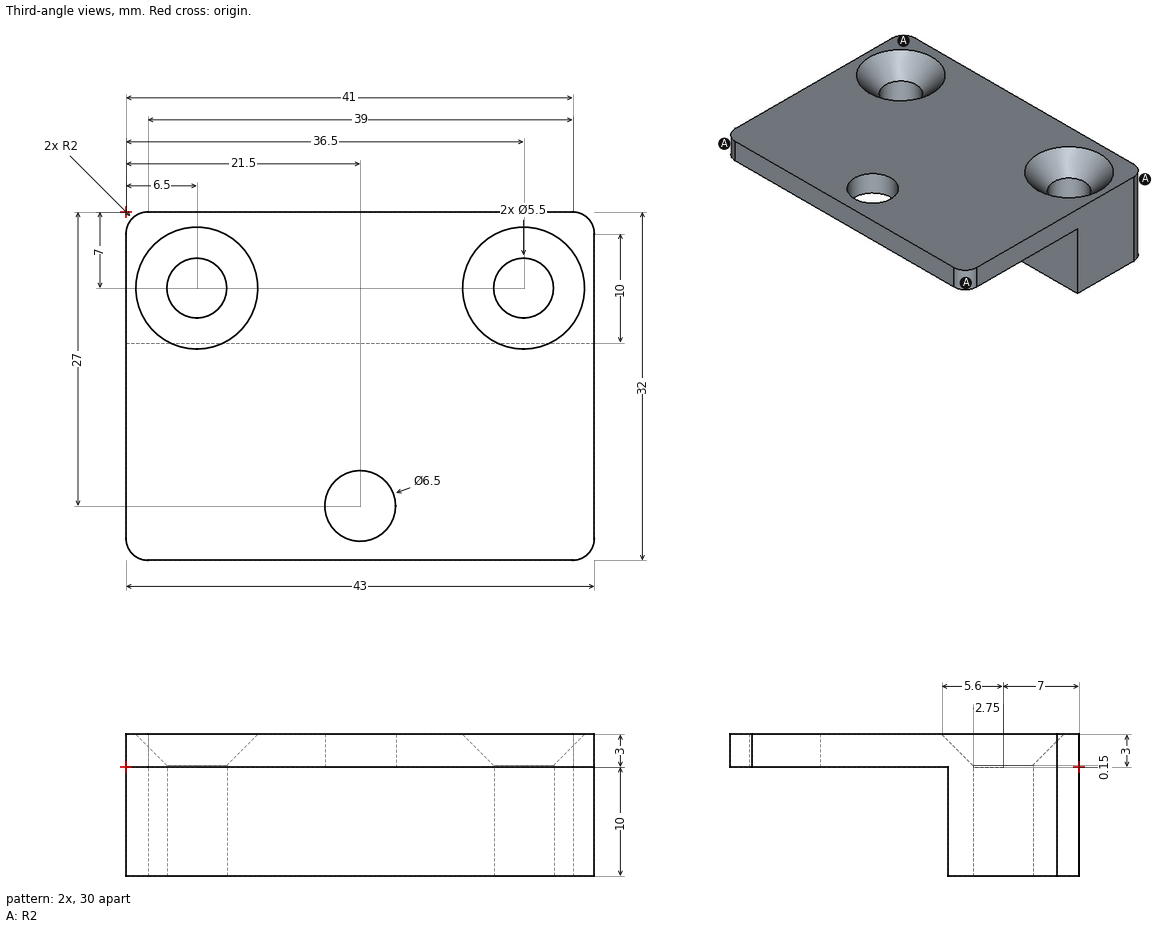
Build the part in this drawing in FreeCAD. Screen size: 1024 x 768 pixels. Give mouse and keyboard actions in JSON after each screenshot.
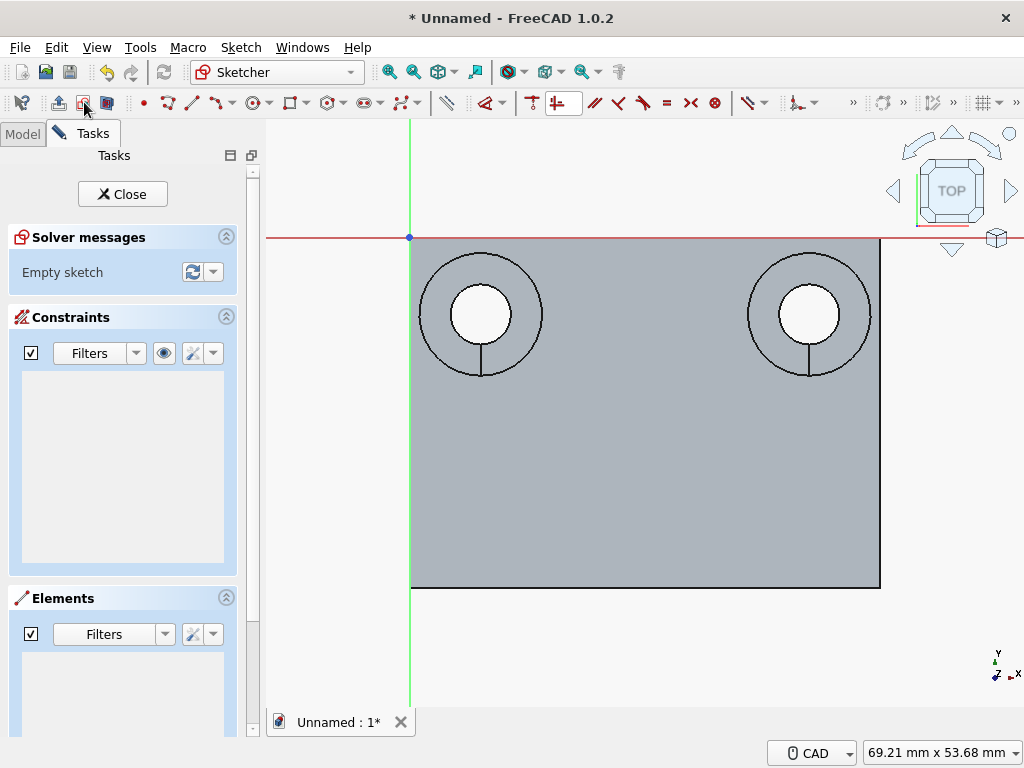
{"action": "scroll", "coordinate": [662, 564], "scroll_direction": "up", "scroll_amount": 8}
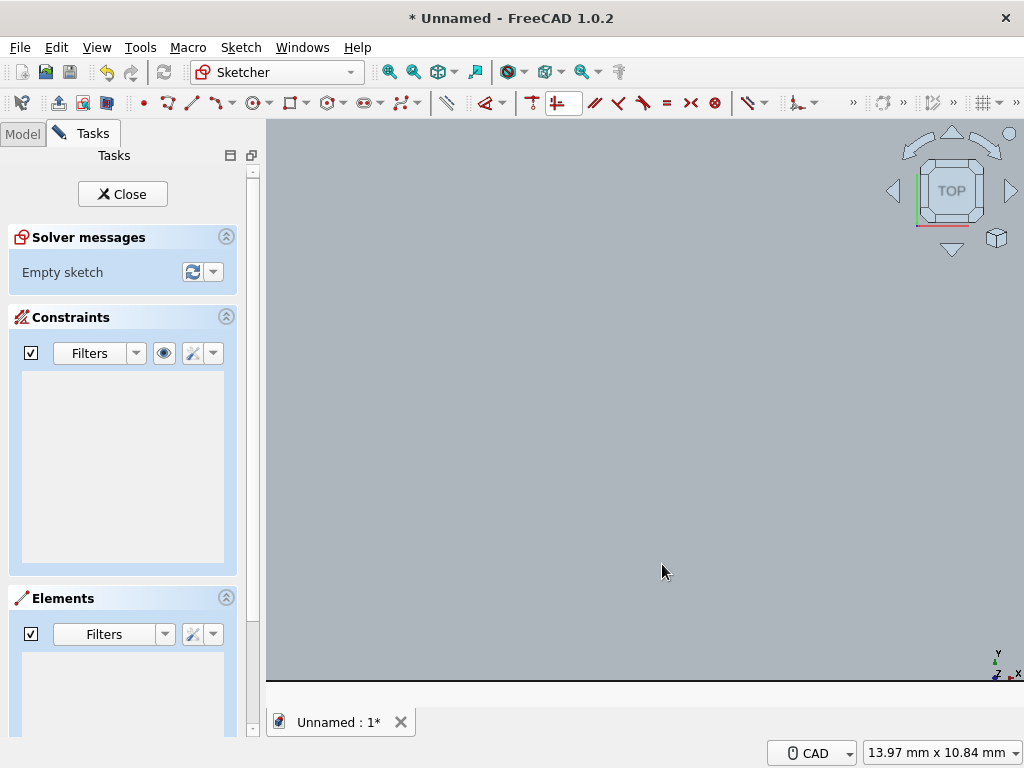
{"action": "key", "text": "g c"}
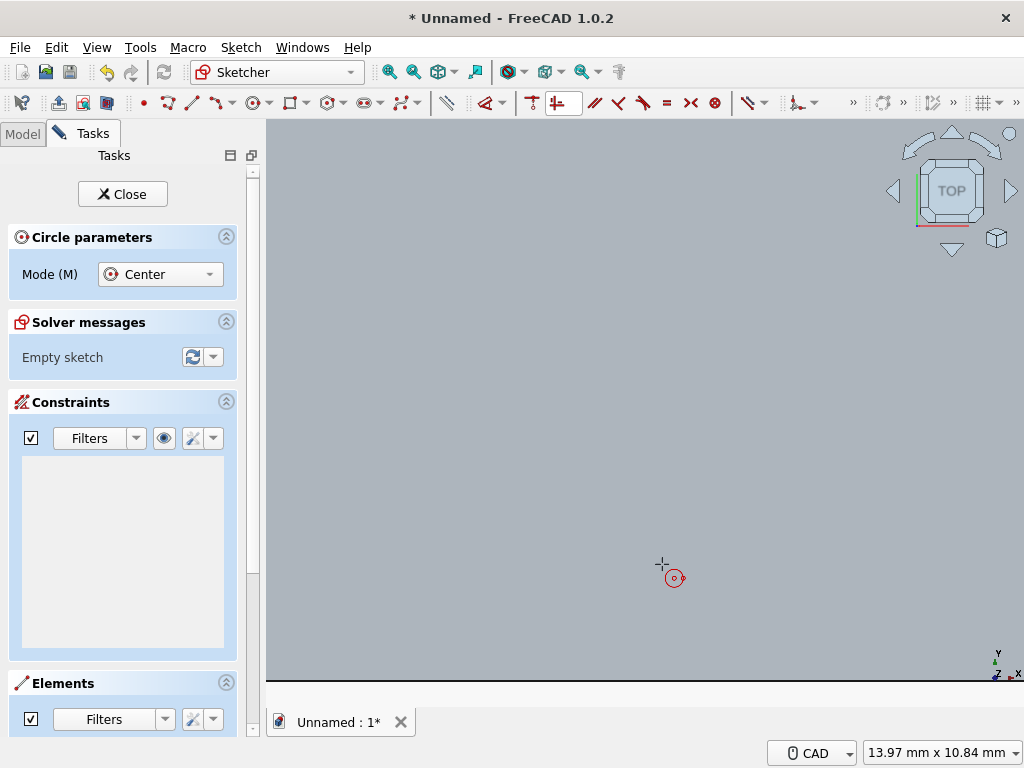
{"action": "left_click", "coordinate": [576, 410]}
{"action": "mouse_move", "coordinate": [700, 285]}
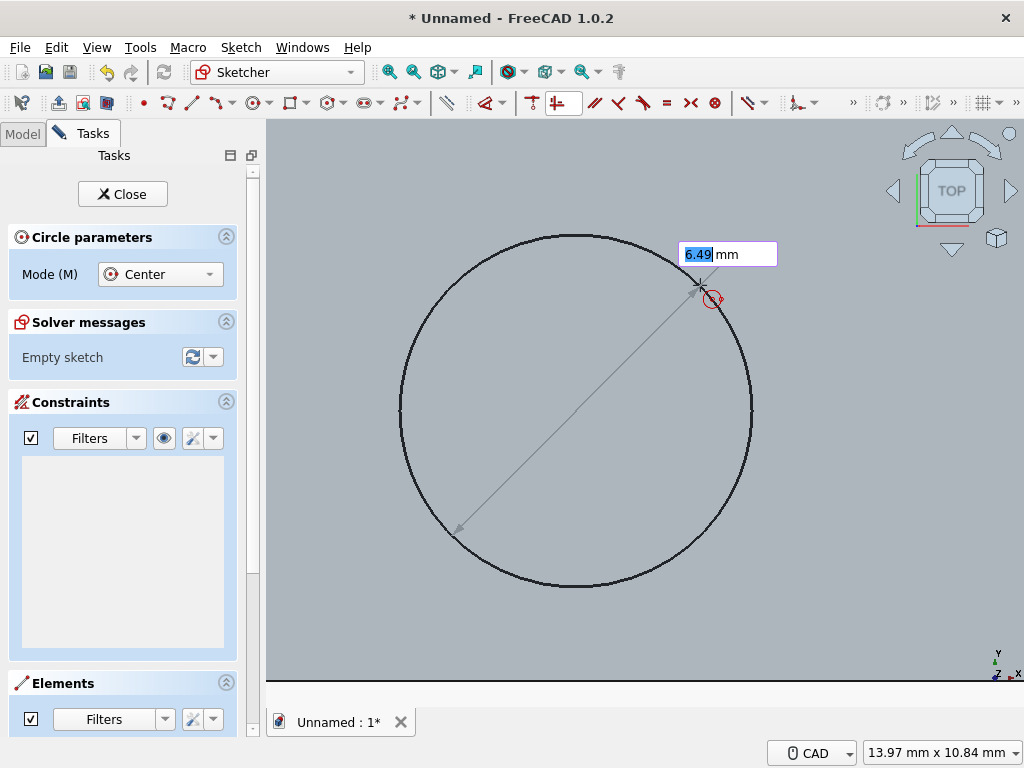
{"action": "type", "text": "6.5"}
{"action": "key", "text": "Return"}
{"action": "key", "text": "Escape"}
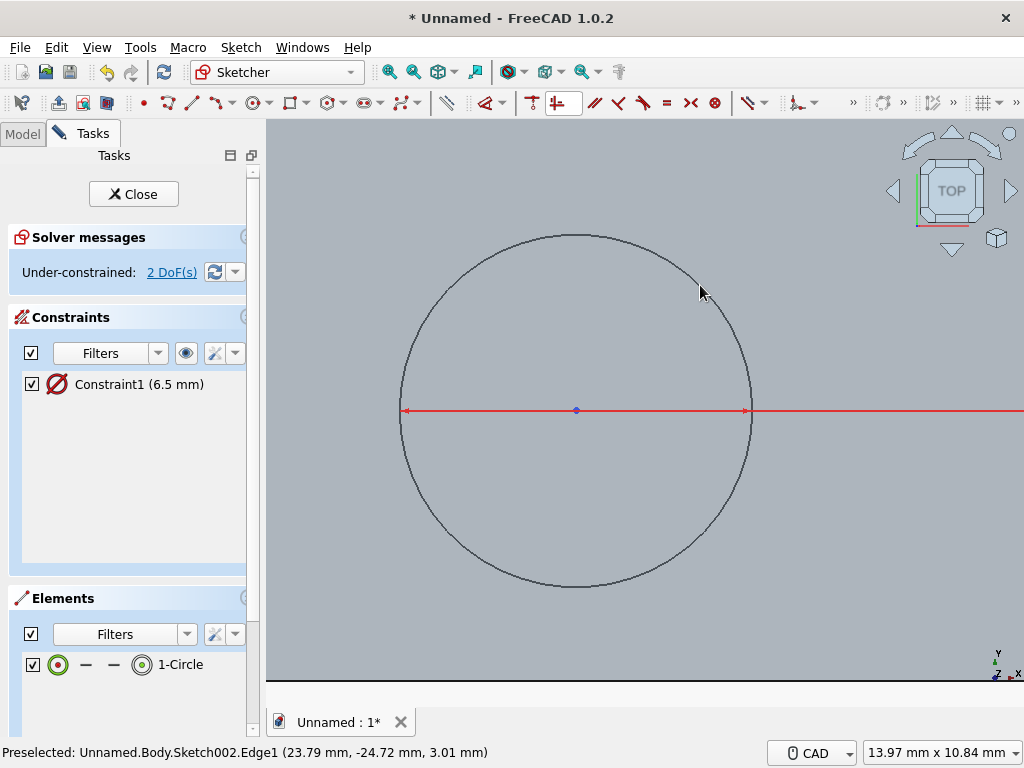
{"action": "key", "text": "d"}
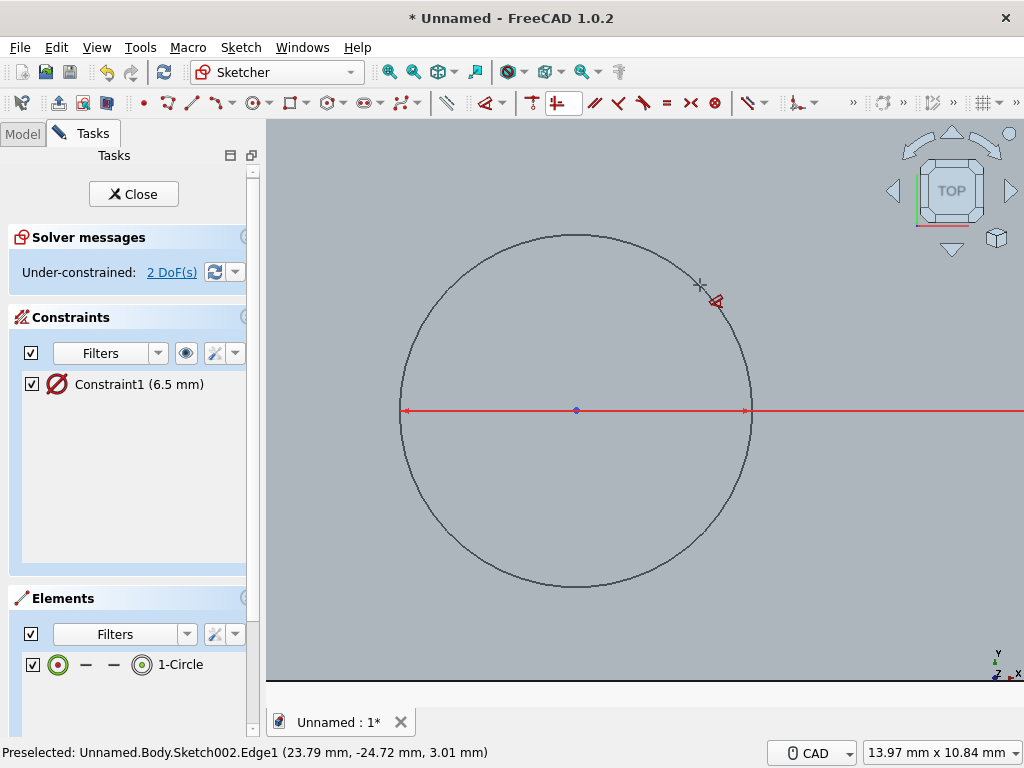
{"action": "left_click", "coordinate": [576, 411]}
{"action": "left_click", "coordinate": [610, 279]}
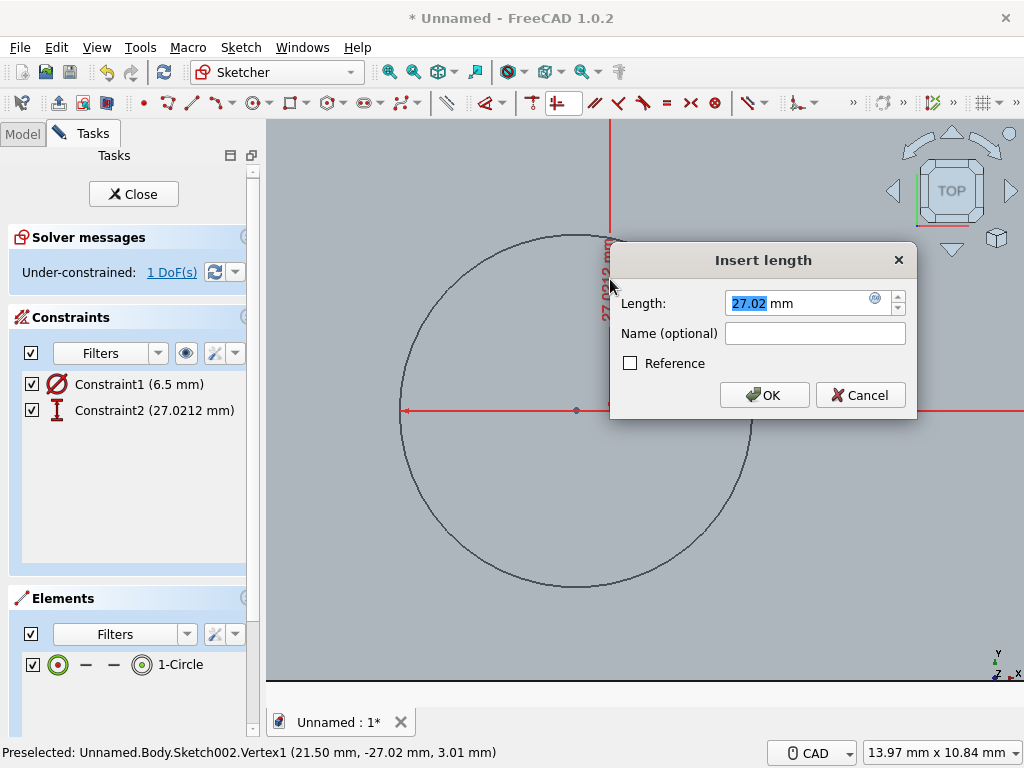
{"action": "type", "text": "27"}
{"action": "key", "text": "Return"}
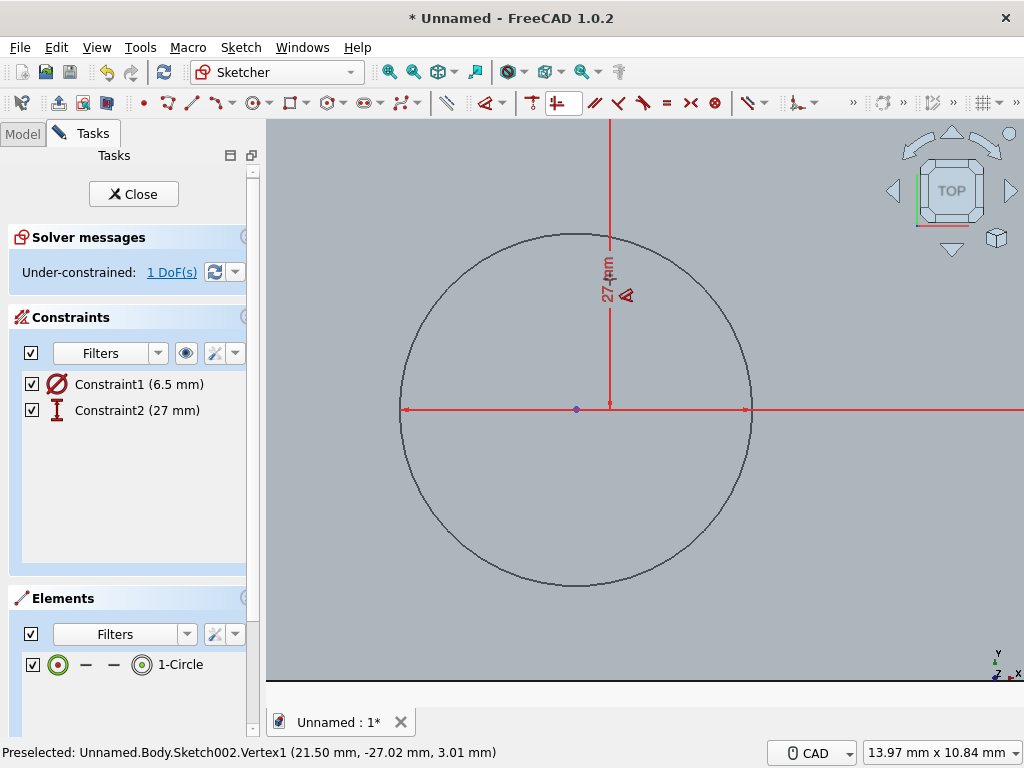
{"action": "left_click", "coordinate": [576, 410]}
{"action": "left_click", "coordinate": [435, 444]}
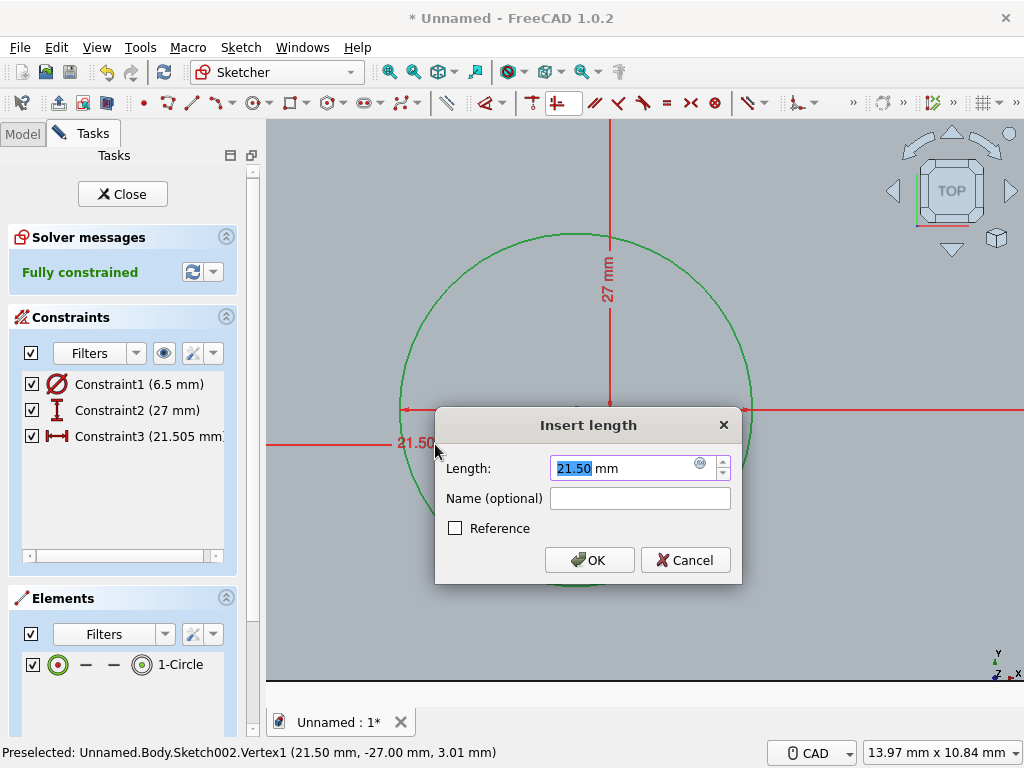
{"action": "type", "text": "21.5"}
{"action": "key", "text": "Return"}
{"action": "key", "text": "Escape"}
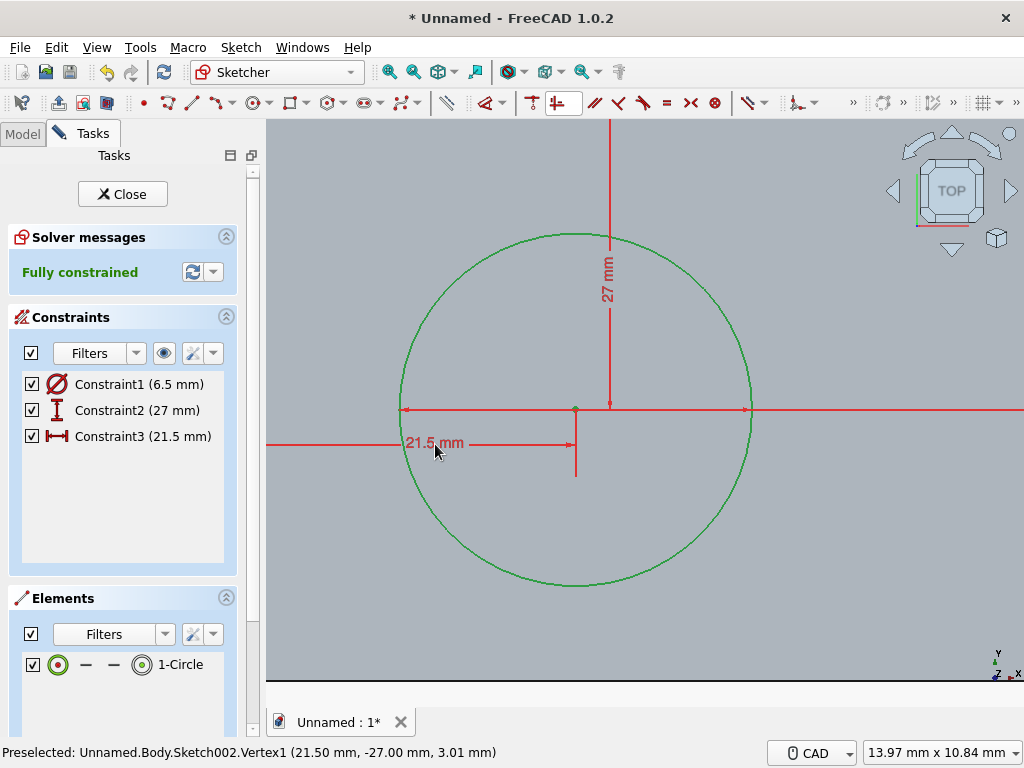
{"action": "left_click", "coordinate": [123, 194]}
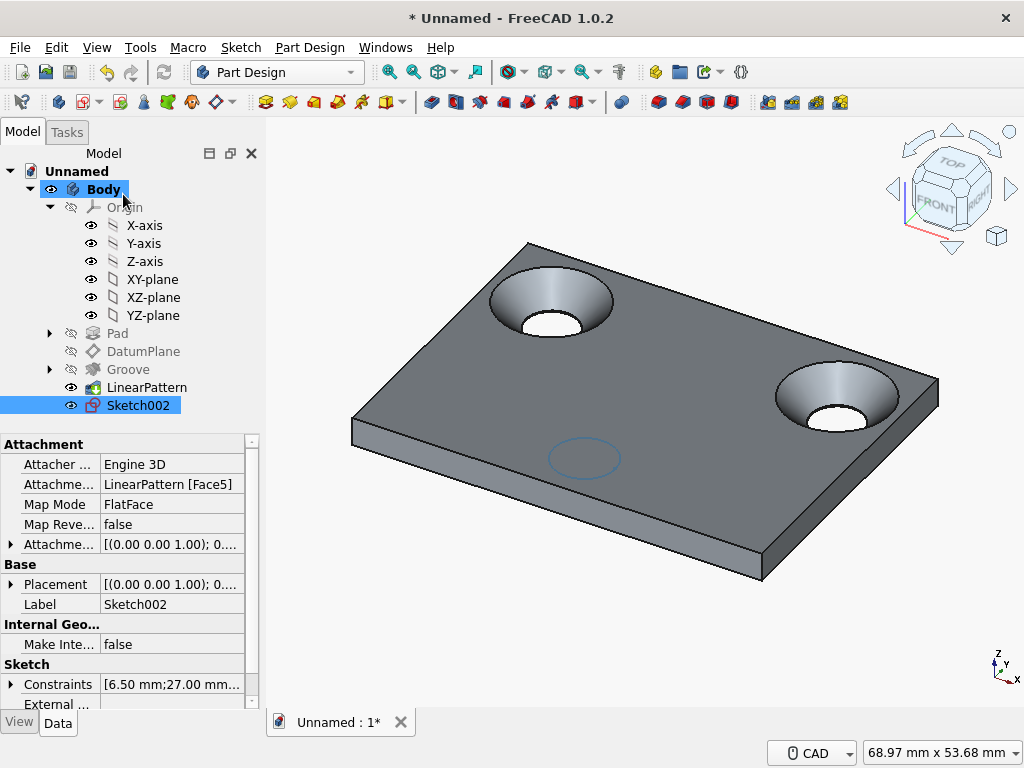
{"action": "left_click", "coordinate": [432, 102]}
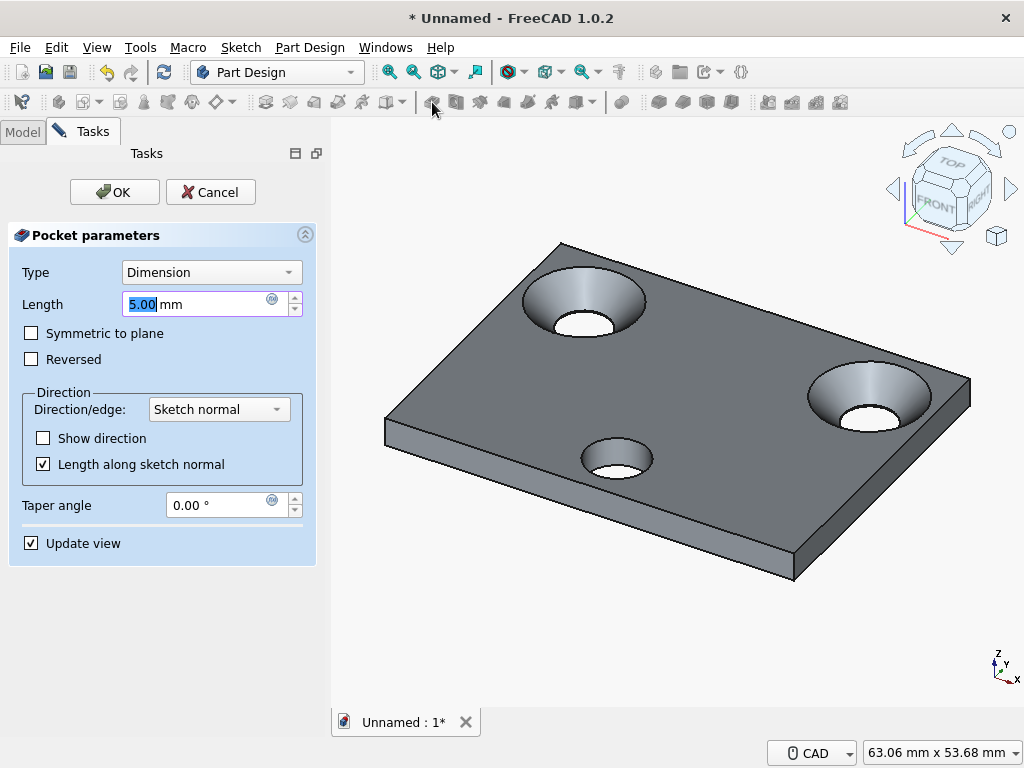
{"action": "type", "text": "3"}
{"action": "key", "text": "Tab"}